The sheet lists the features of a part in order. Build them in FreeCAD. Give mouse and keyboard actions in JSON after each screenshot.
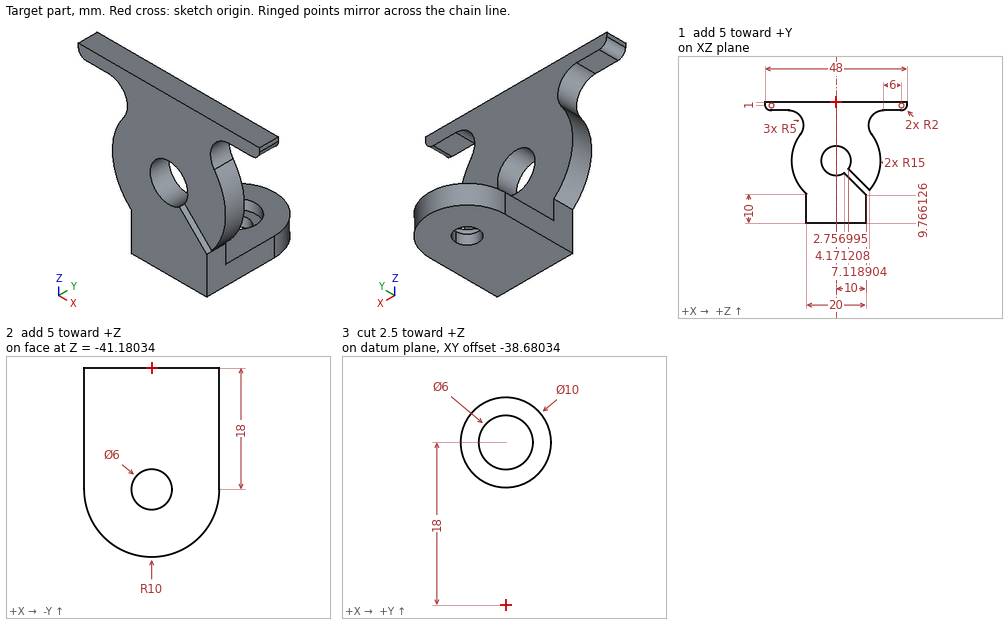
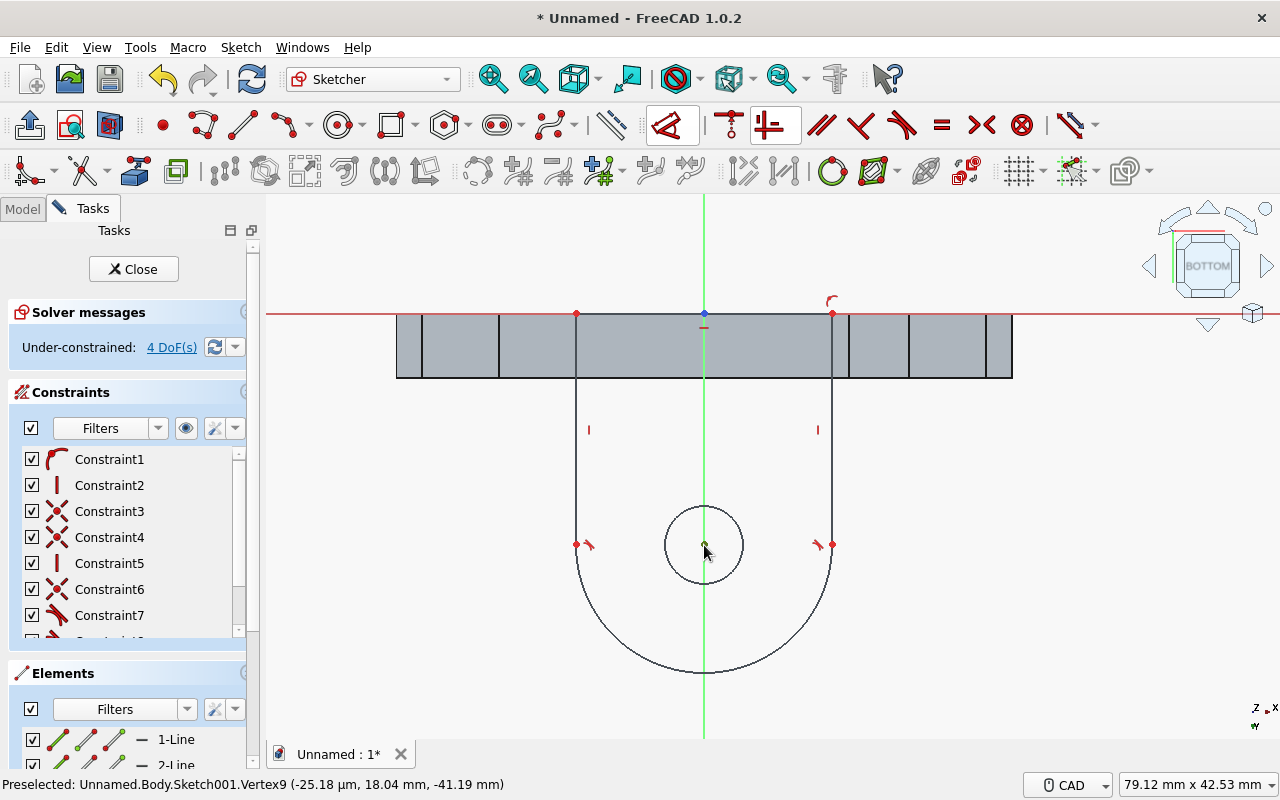
{"action": "left_click", "coordinate": [704, 641]}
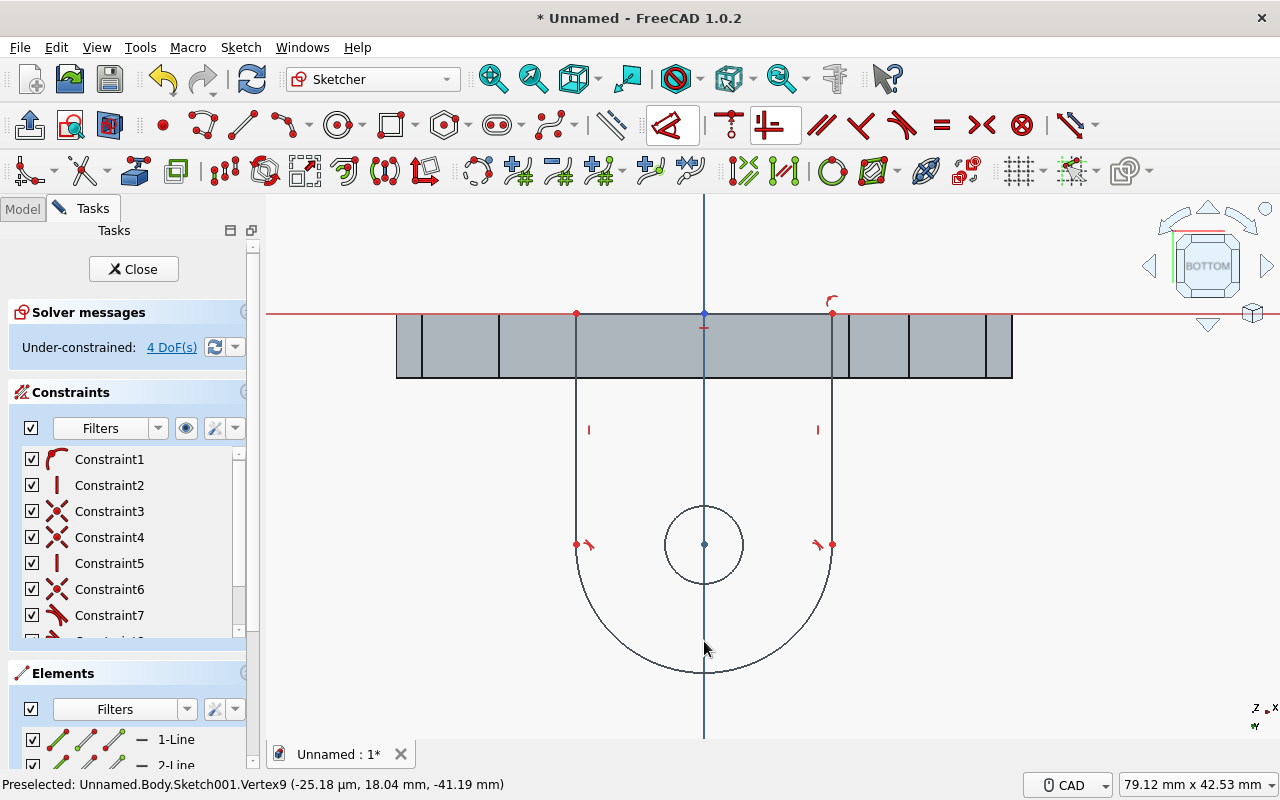
{"action": "key", "text": "c"}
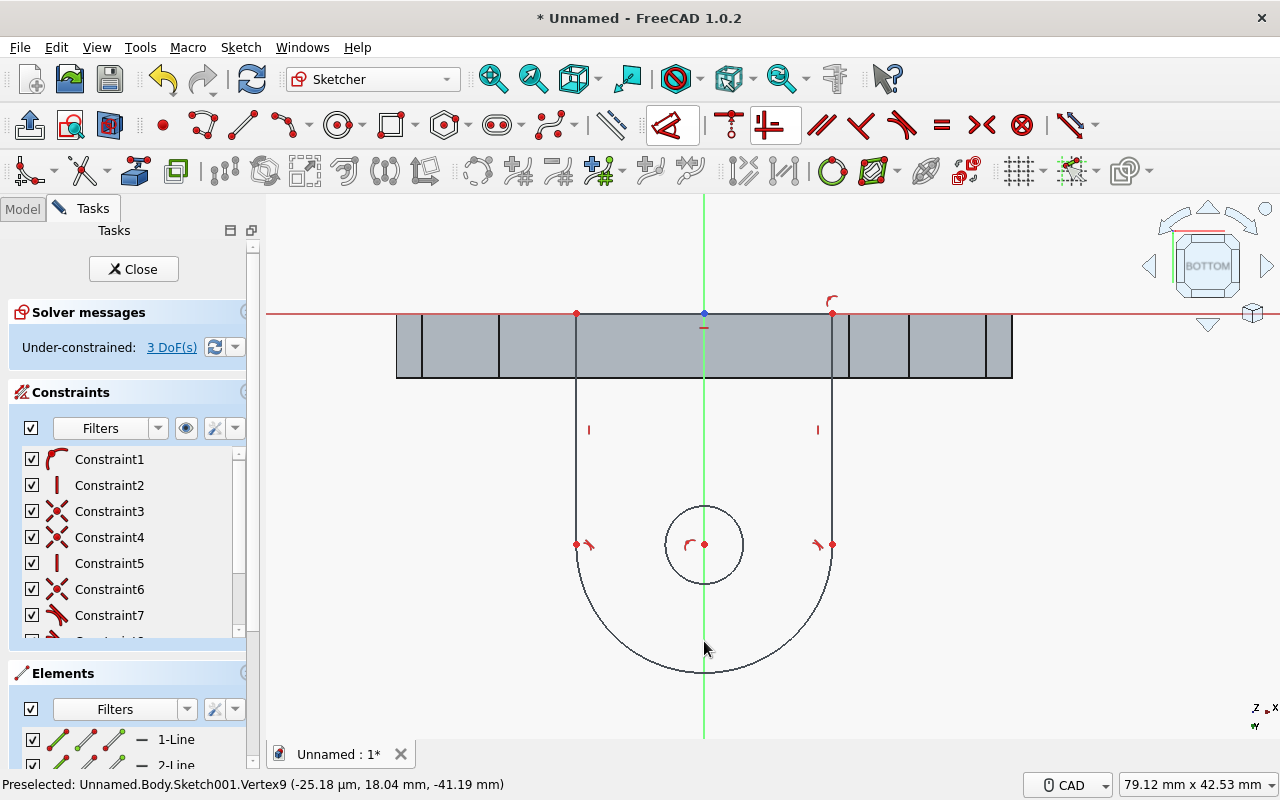
{"action": "left_click", "coordinate": [629, 649]}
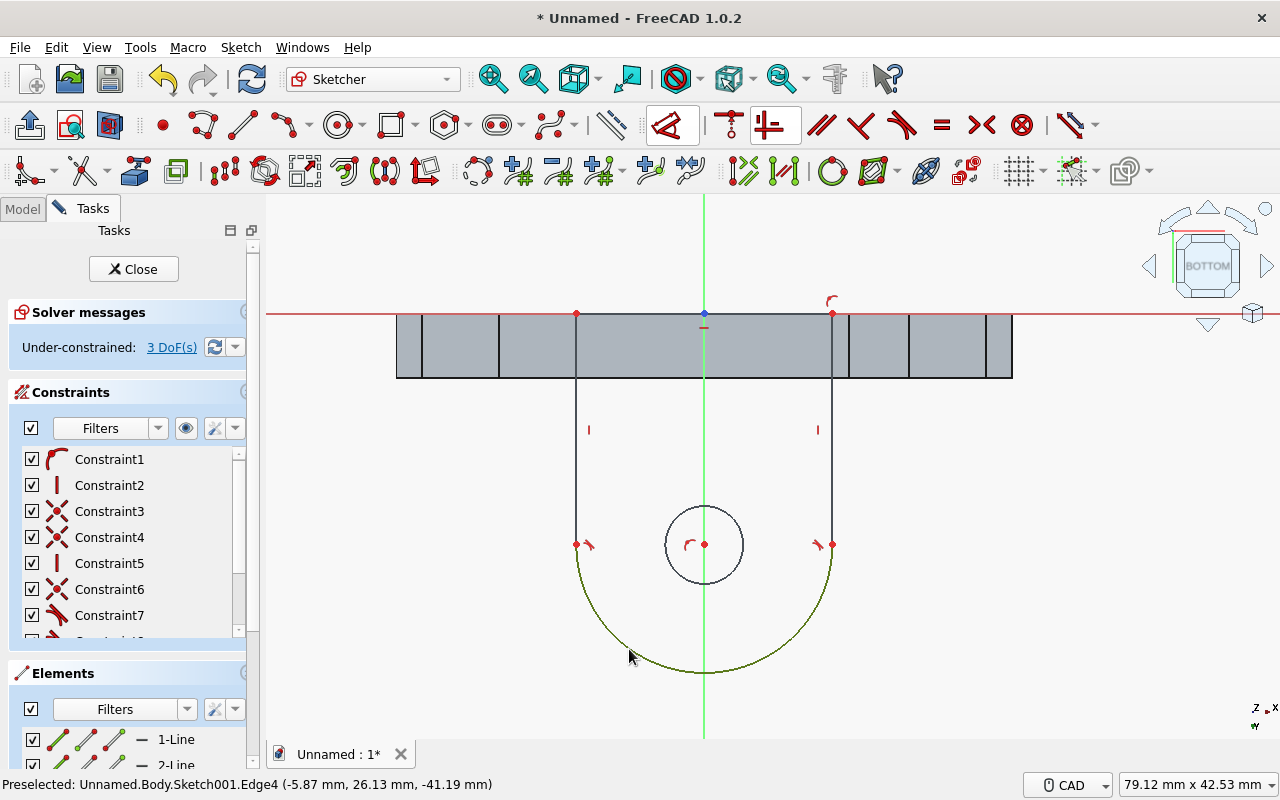
{"action": "key", "text": "k r"}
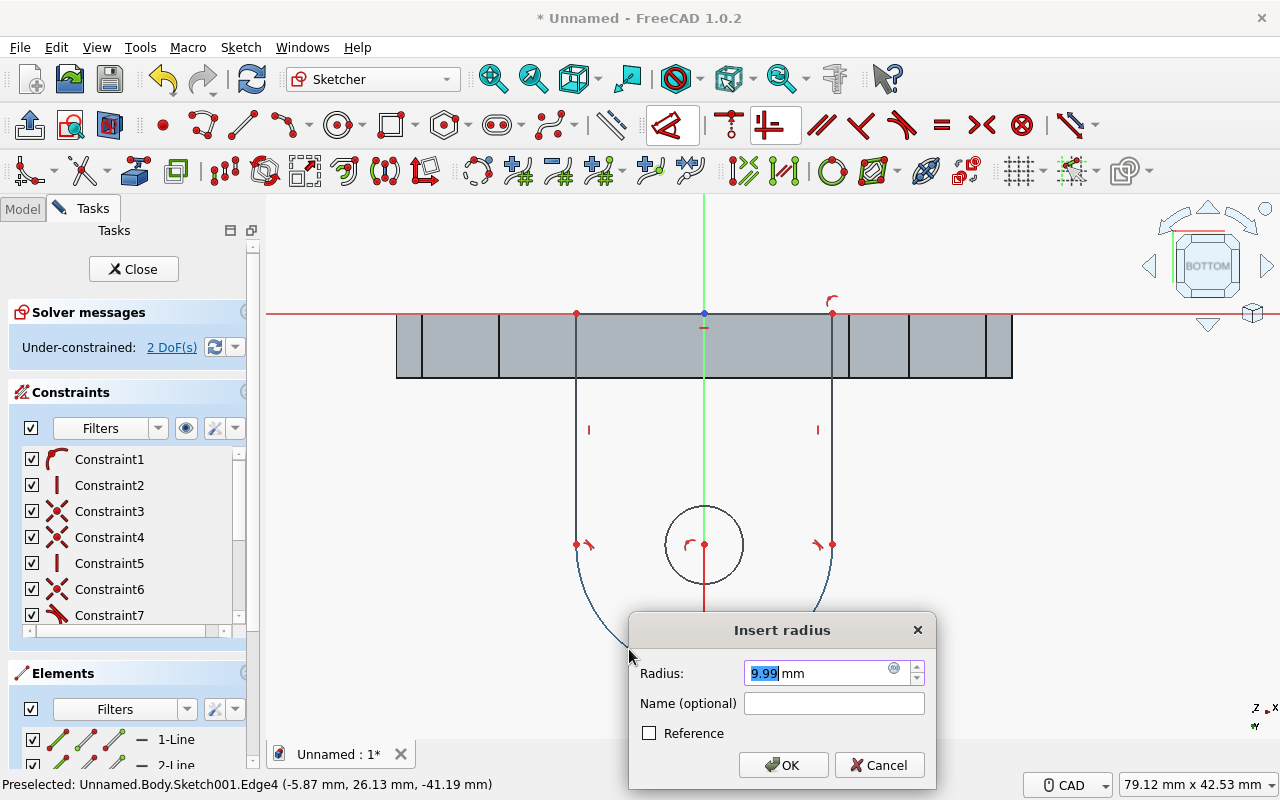
{"action": "type", "text": "10"}
{"action": "key", "text": "Return"}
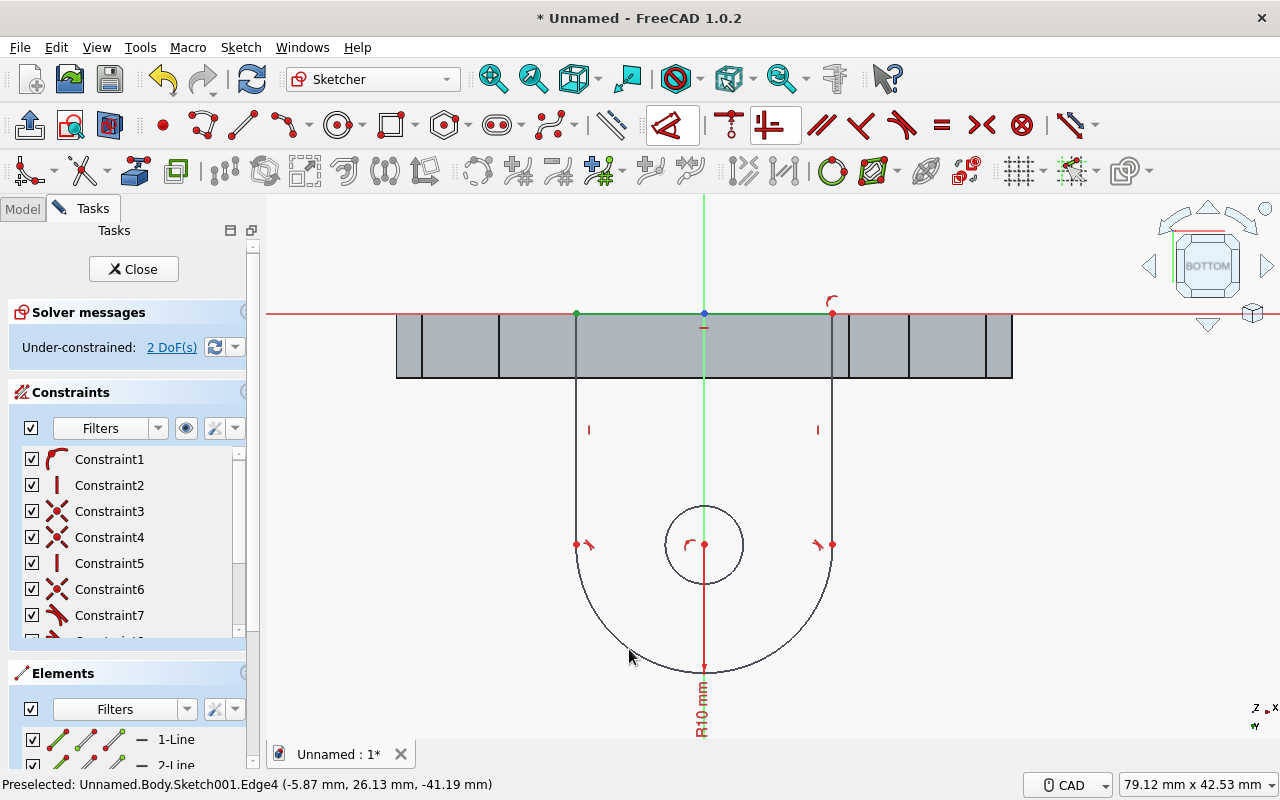
{"action": "left_click", "coordinate": [732, 517]}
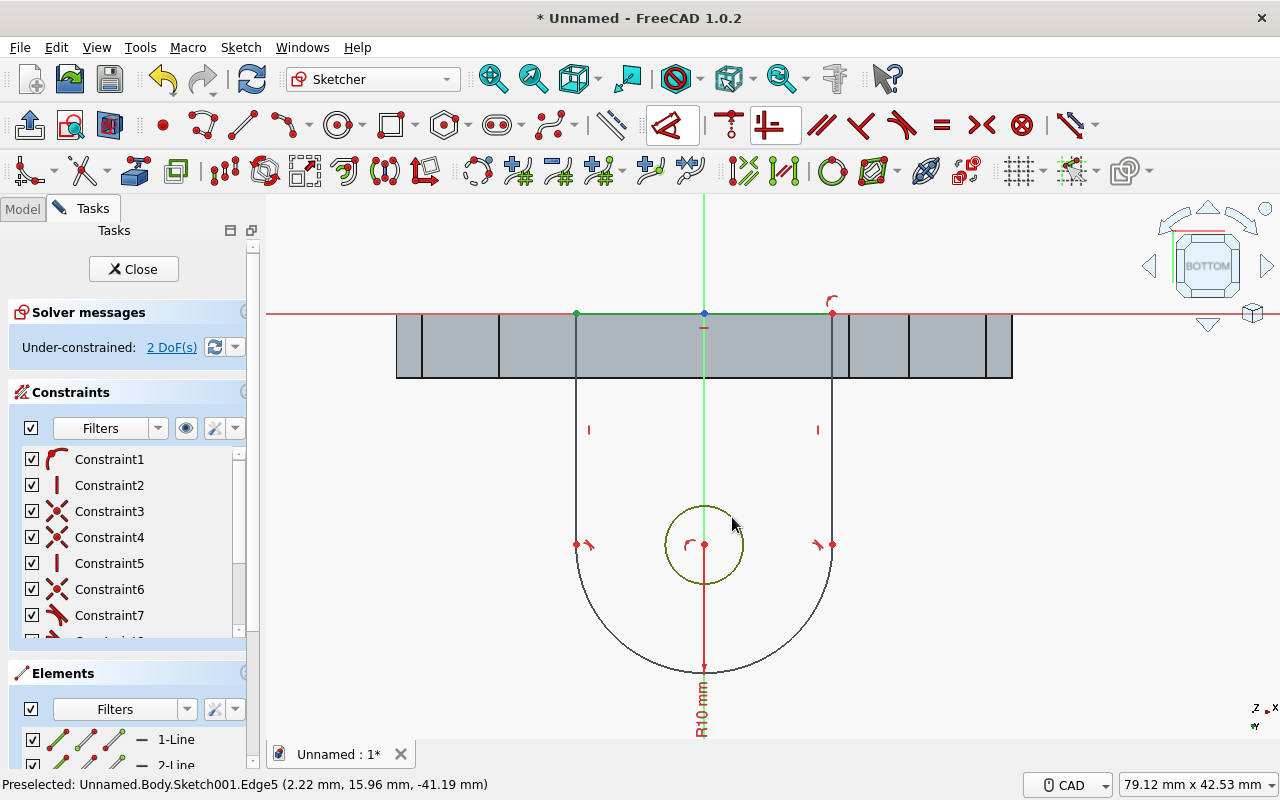
{"action": "key", "text": "k o"}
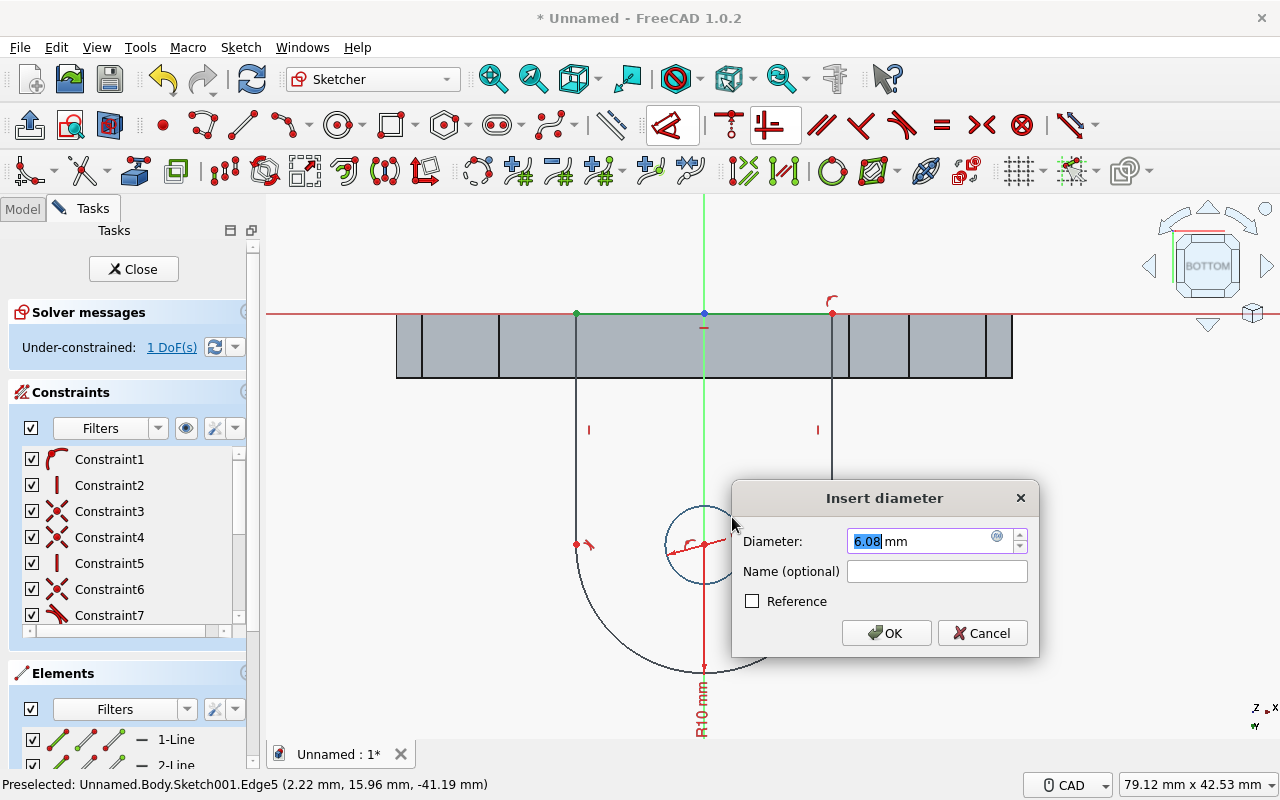
{"action": "type", "text": "6"}
{"action": "key", "text": "Return"}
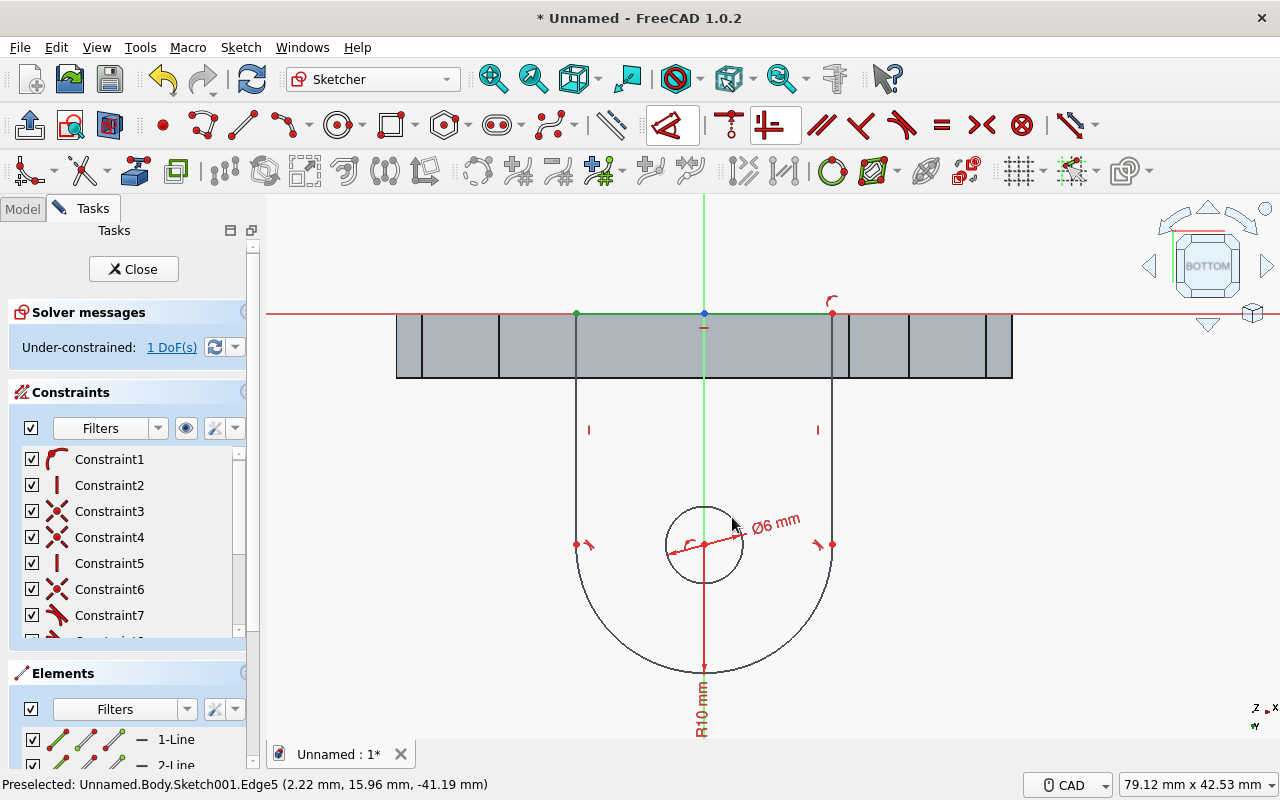
{"action": "left_click", "coordinate": [832, 476]}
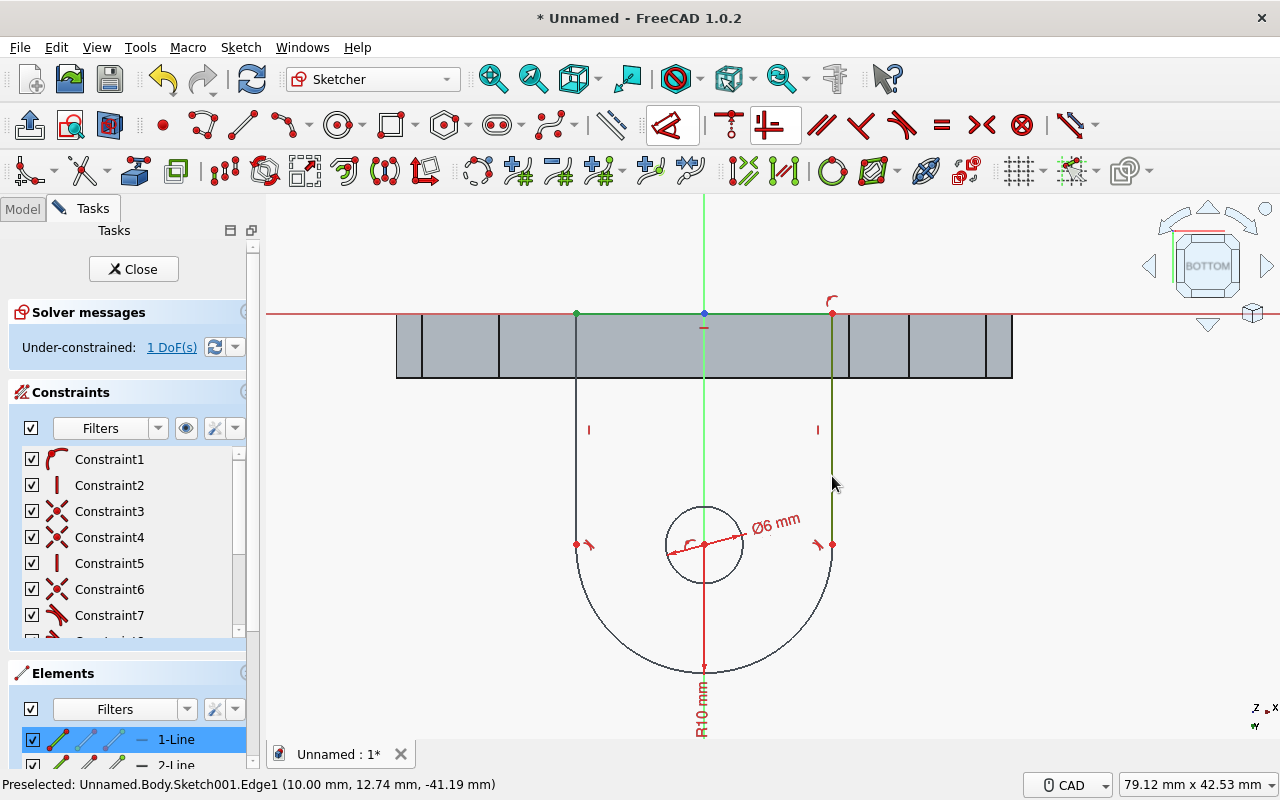
{"action": "key", "text": "i"}